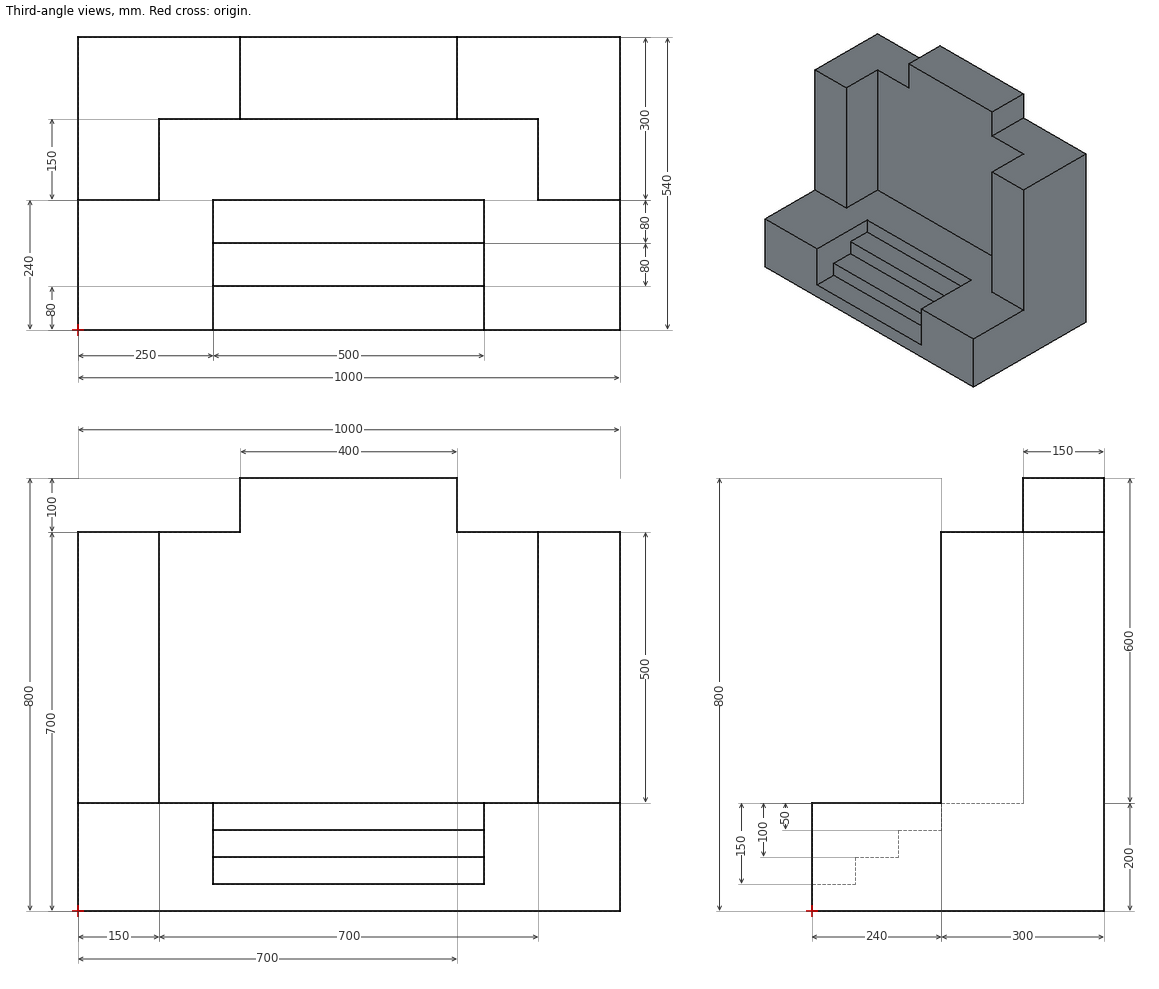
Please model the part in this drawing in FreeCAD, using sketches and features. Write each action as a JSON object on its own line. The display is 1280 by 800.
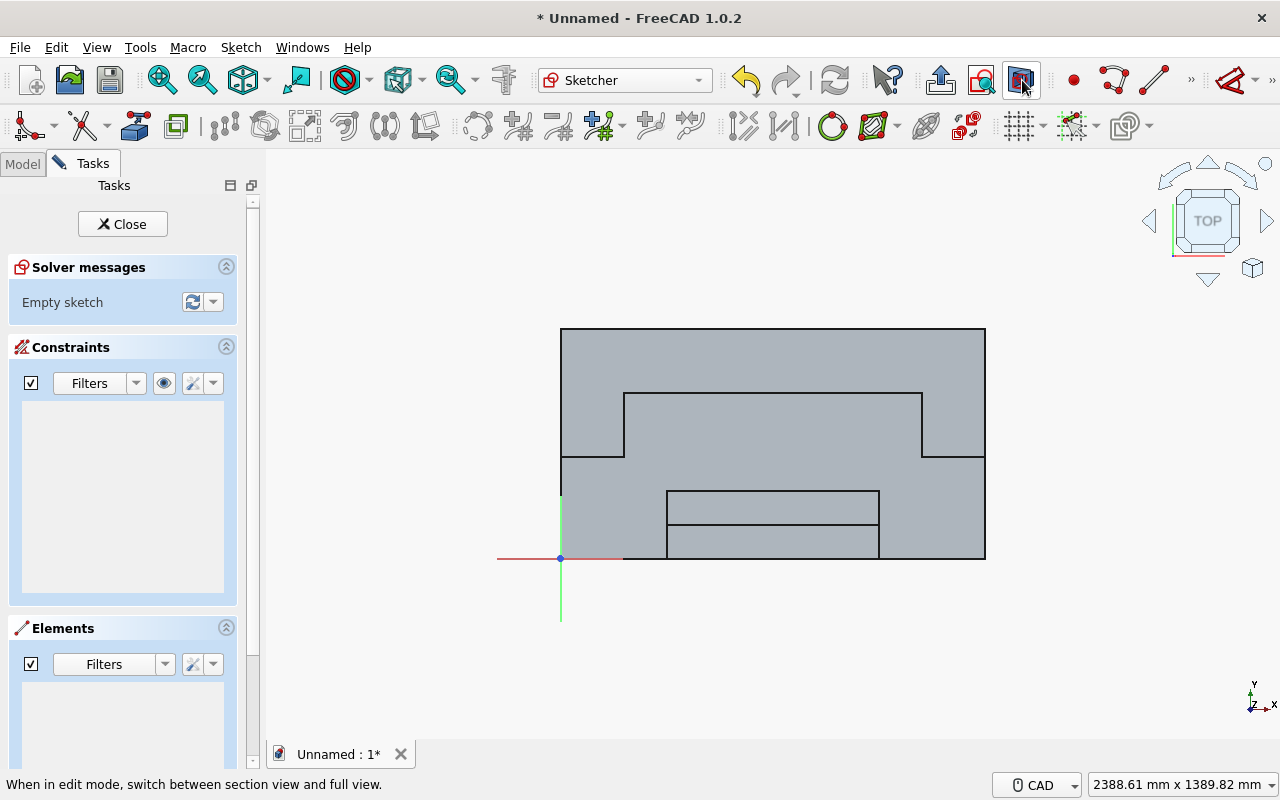
{"action": "scroll", "coordinate": [739, 585], "scroll_direction": "up", "scroll_amount": 3}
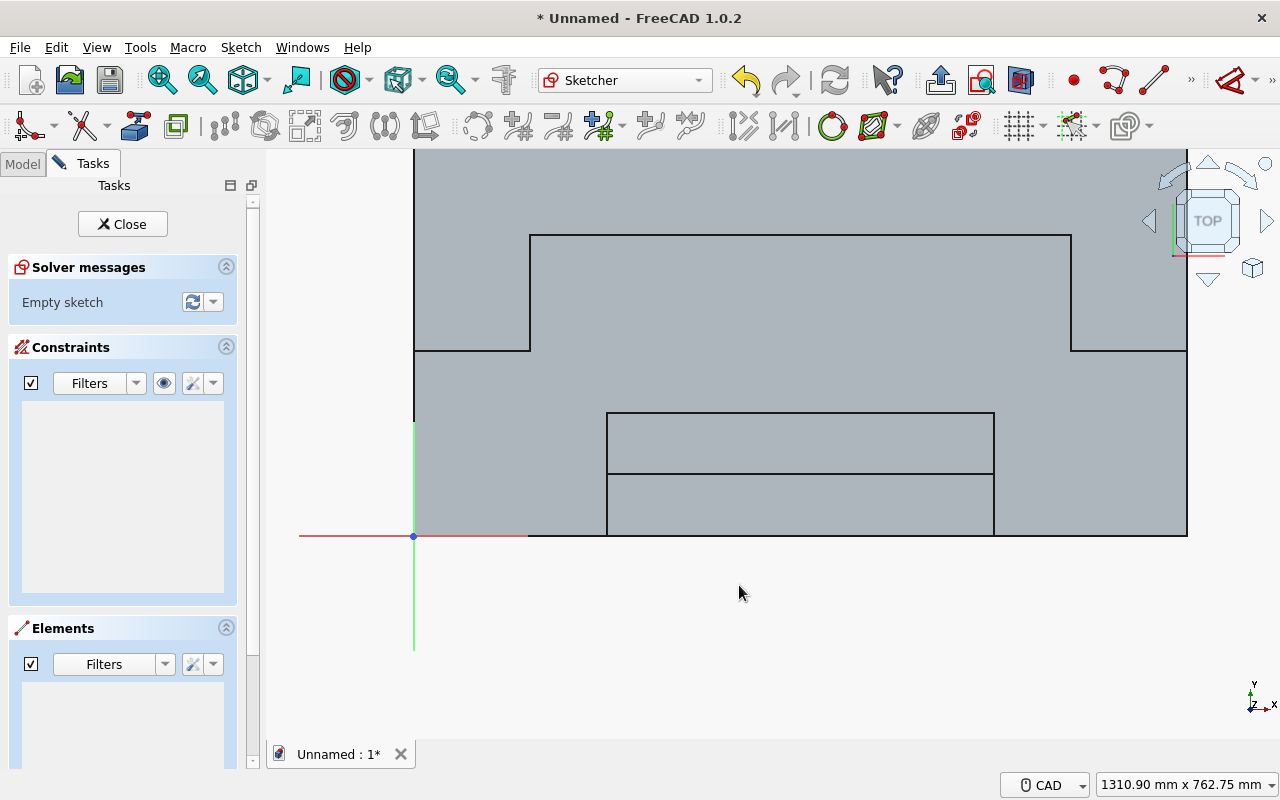
{"action": "key", "text": "g r"}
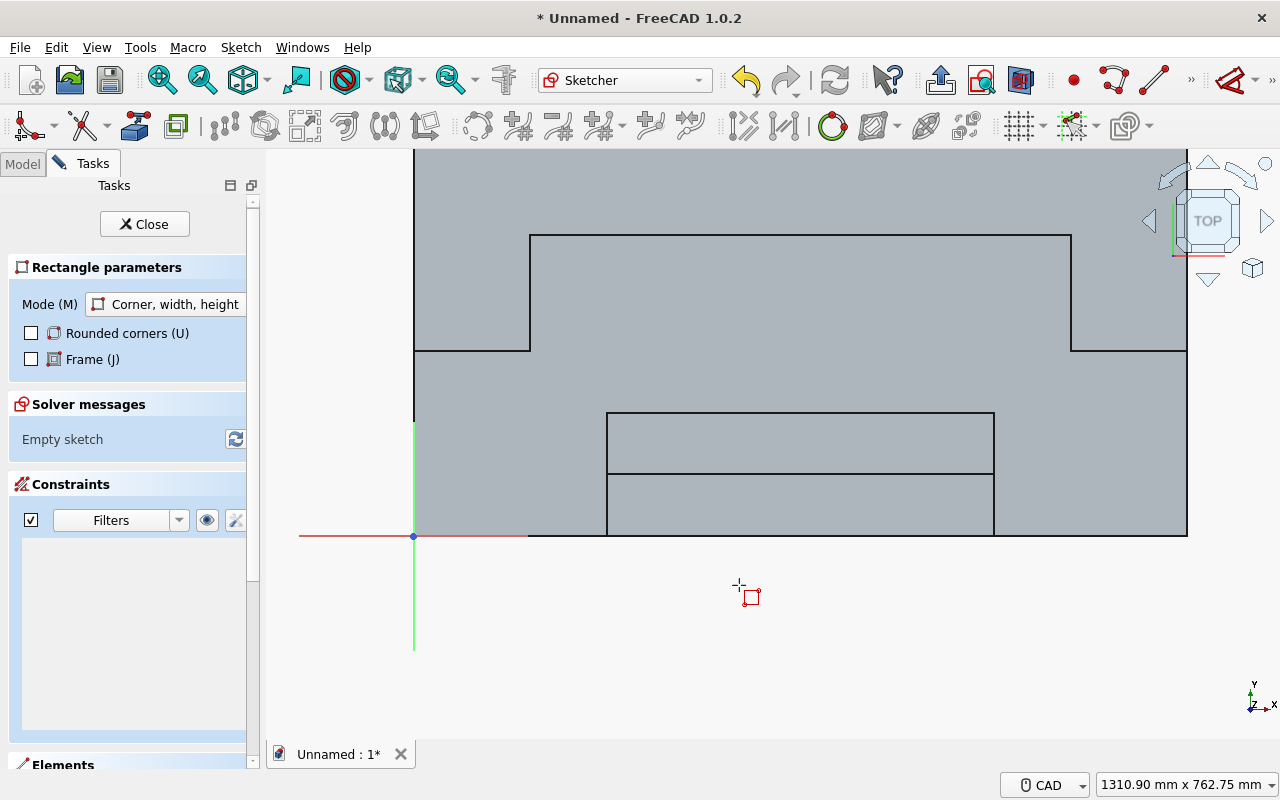
{"action": "left_click", "coordinate": [607, 351]}
{"action": "mouse_move", "coordinate": [994, 413]}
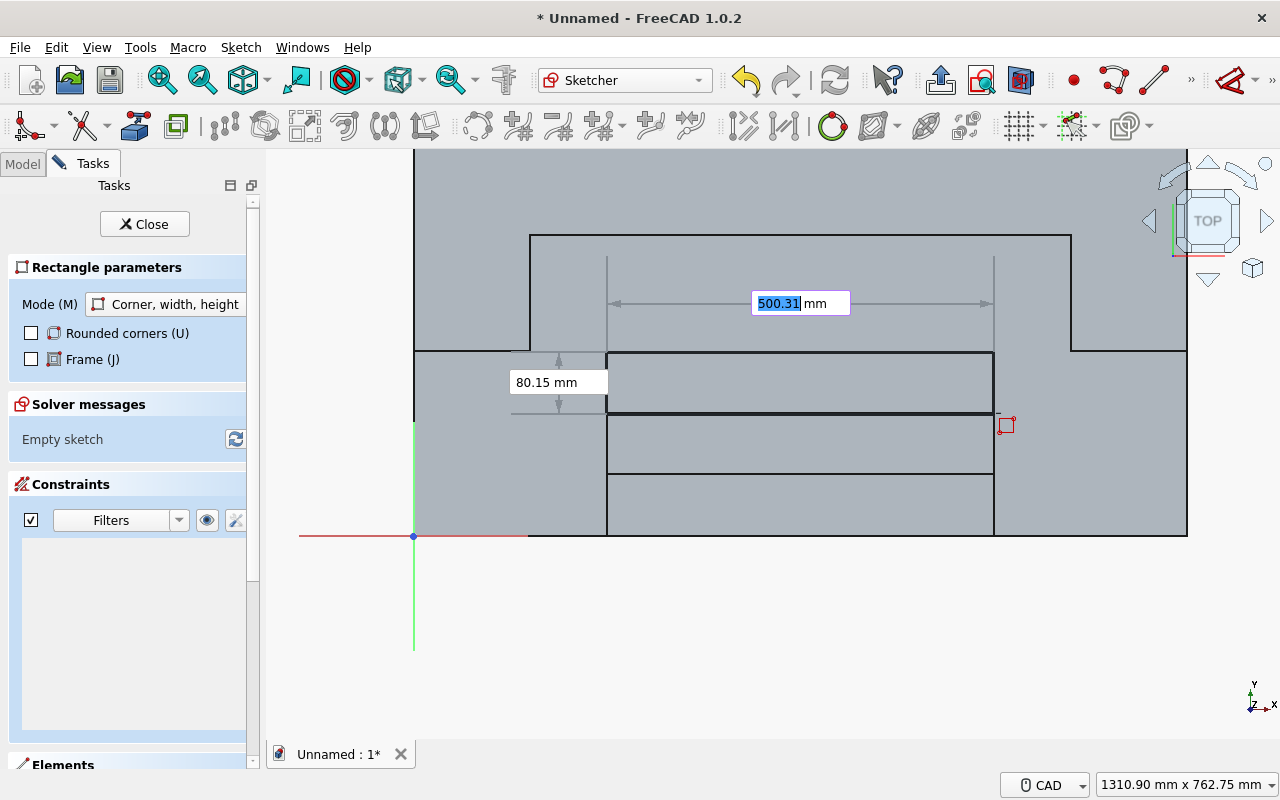
{"action": "type", "text": "500"}
{"action": "key", "text": "Tab"}
{"action": "type", "text": "80"}
{"action": "key", "text": "Return"}
{"action": "key", "text": "Escape"}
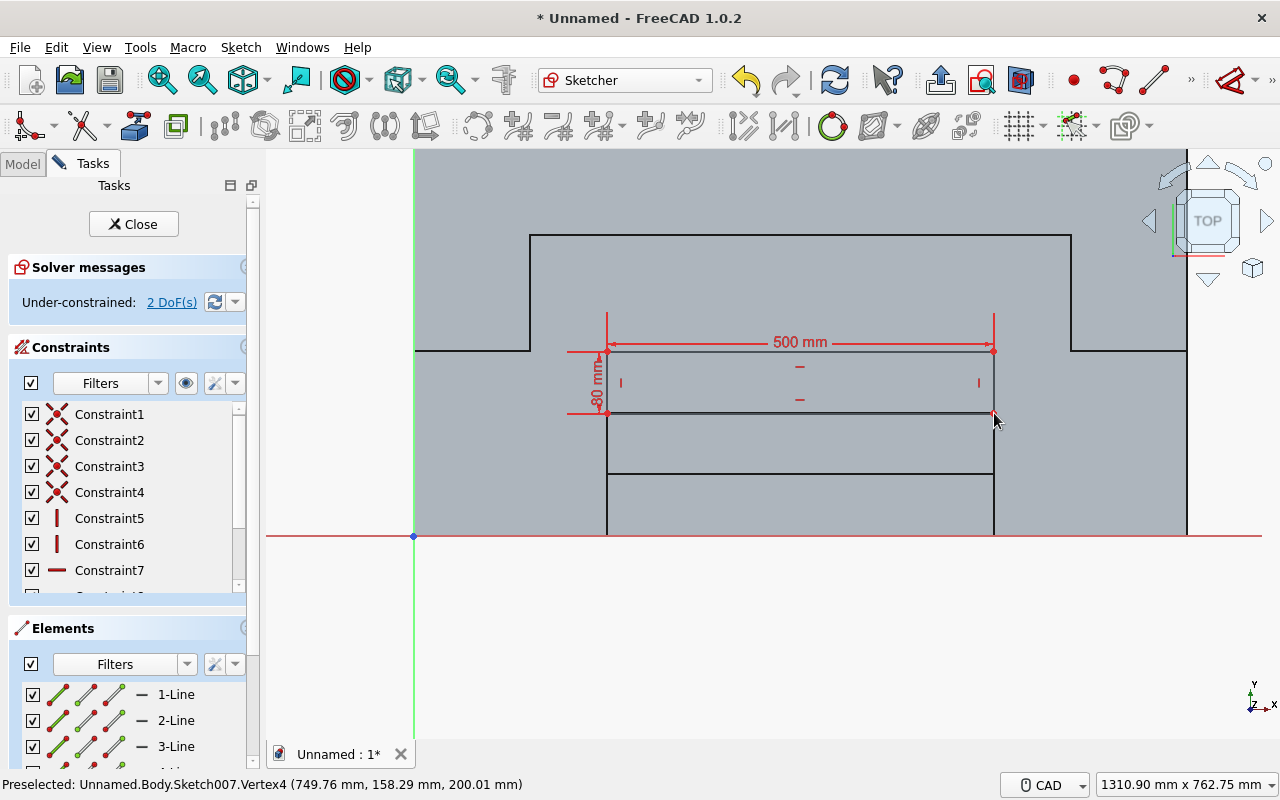
{"action": "left_click", "coordinate": [1230, 80]}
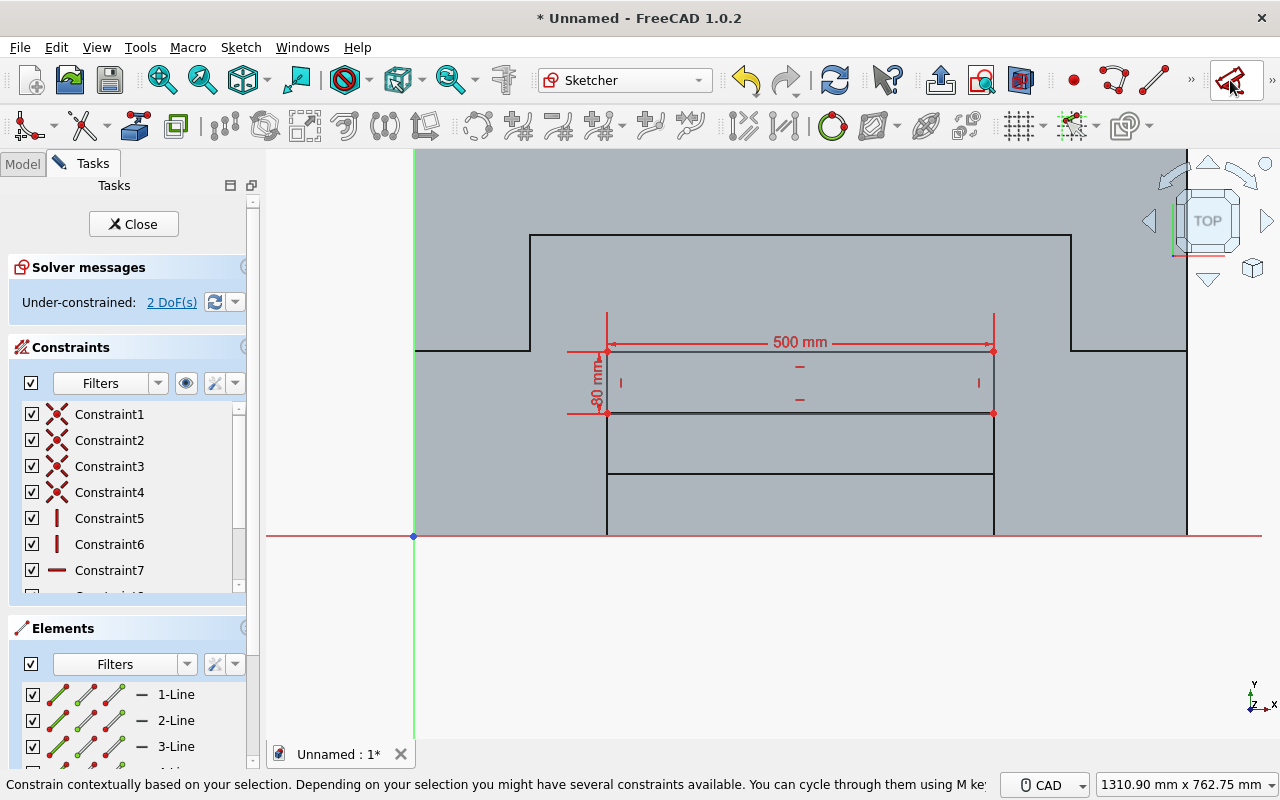
{"action": "left_click", "coordinate": [607, 352]}
{"action": "left_click", "coordinate": [510, 570]}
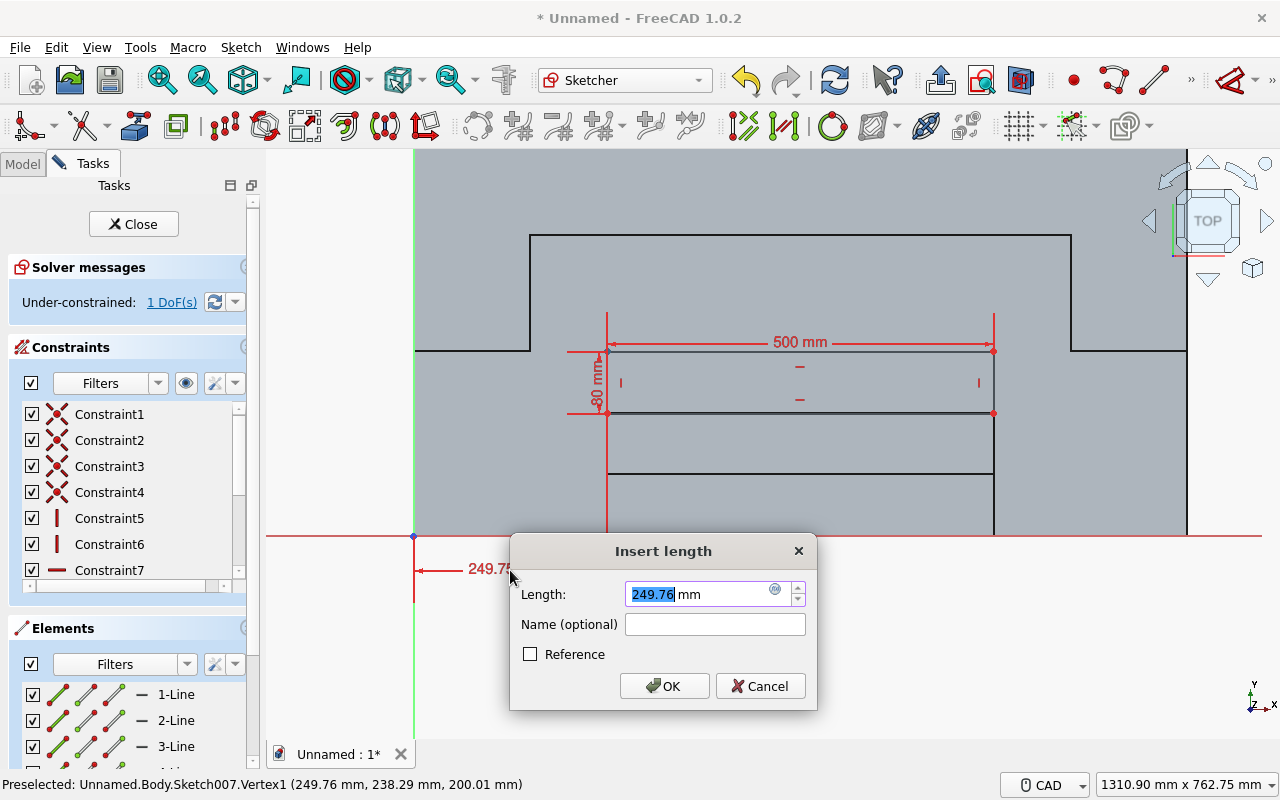
{"action": "type", "text": "250"}
{"action": "key", "text": "Return"}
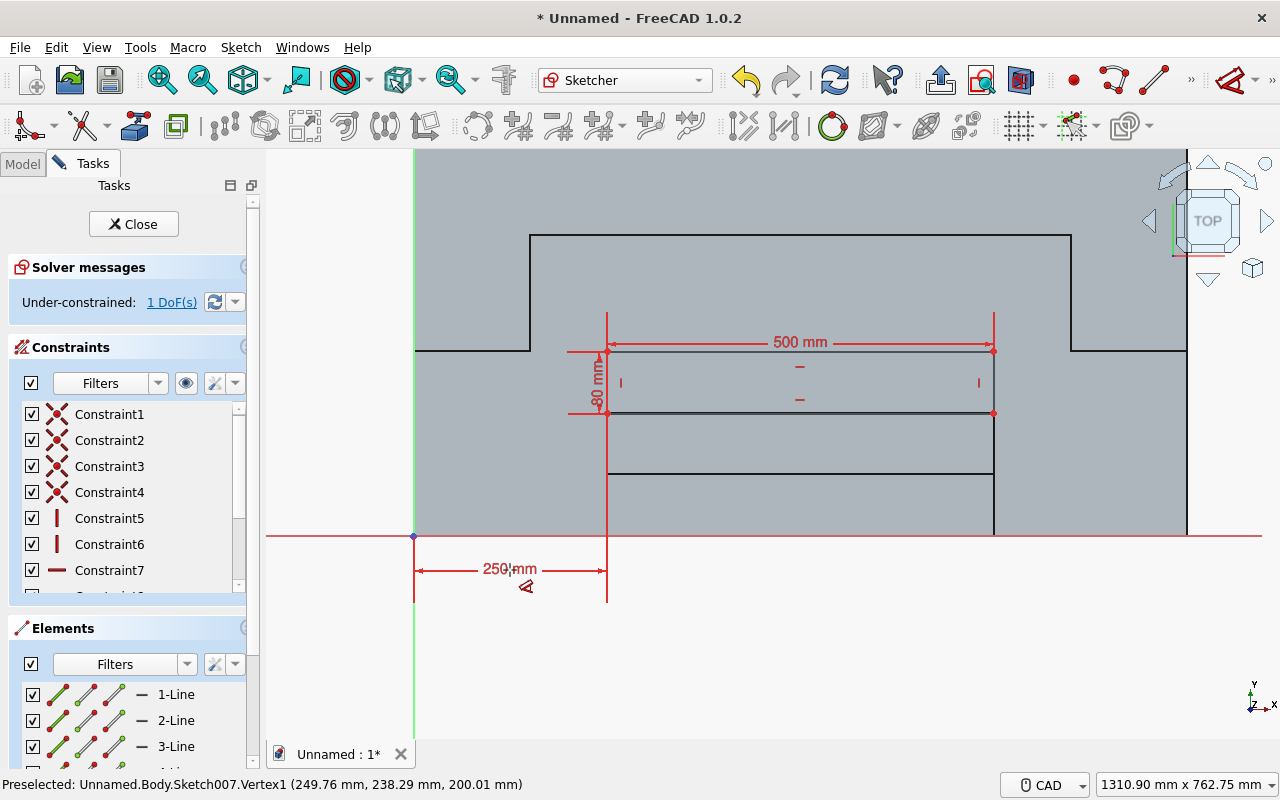
{"action": "left_click", "coordinate": [607, 352]}
{"action": "left_click", "coordinate": [380, 444]}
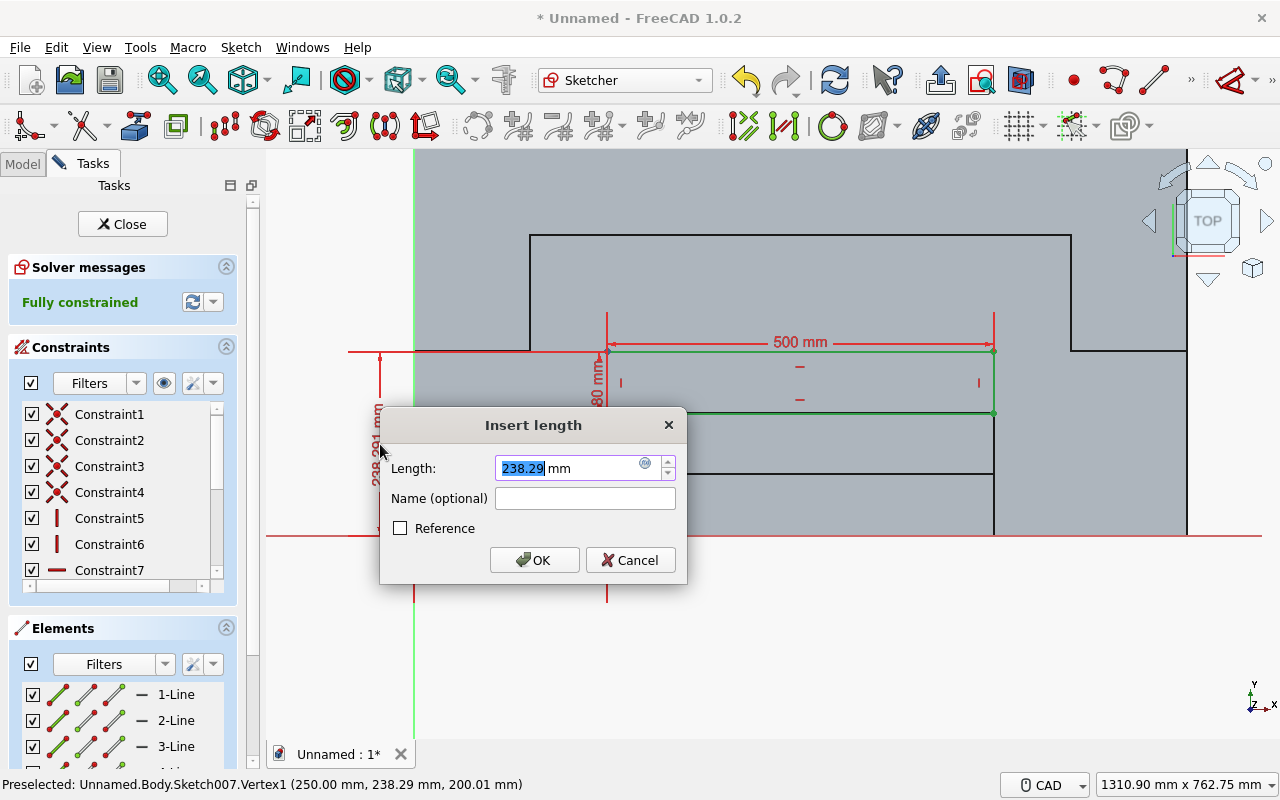
{"action": "type", "text": "240"}
{"action": "key", "text": "Return"}
{"action": "key", "text": "Escape"}